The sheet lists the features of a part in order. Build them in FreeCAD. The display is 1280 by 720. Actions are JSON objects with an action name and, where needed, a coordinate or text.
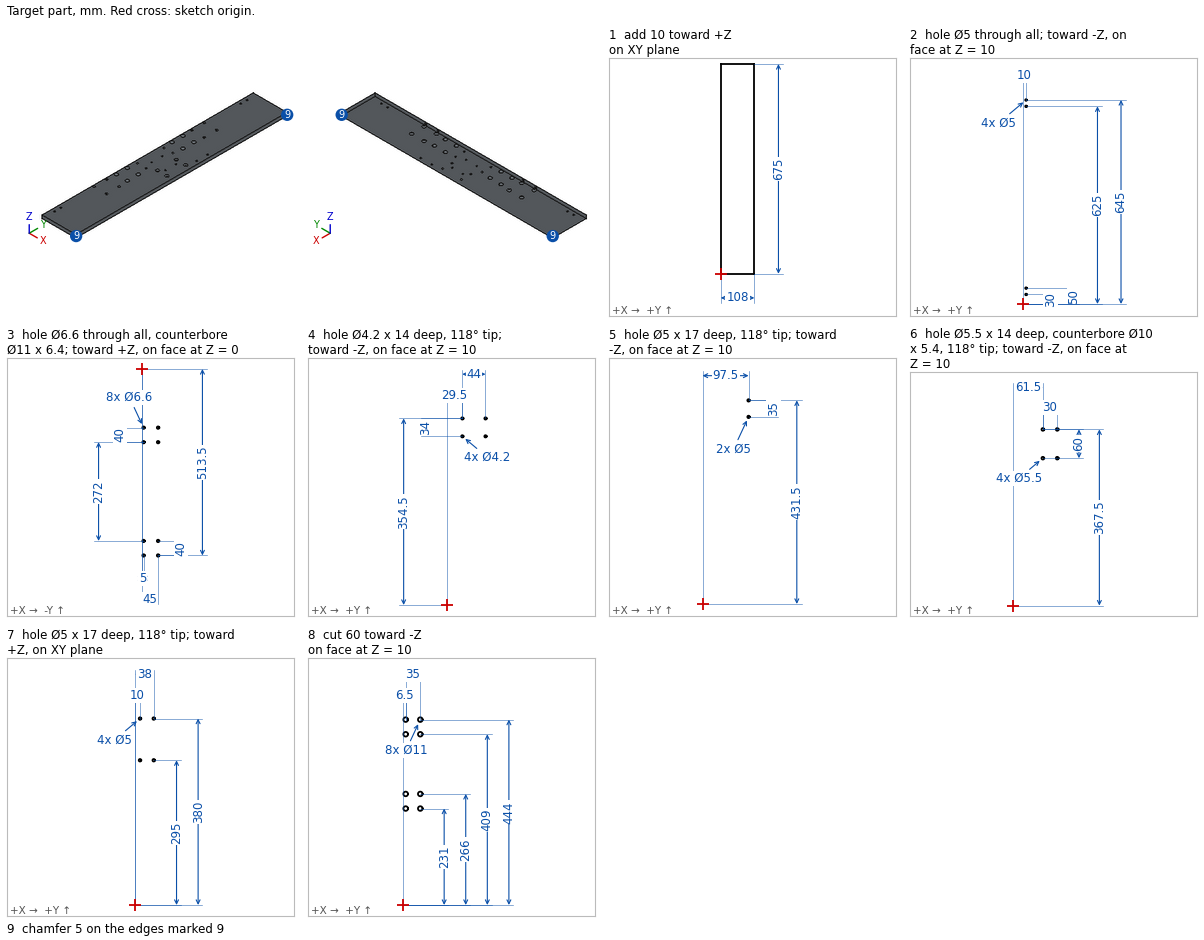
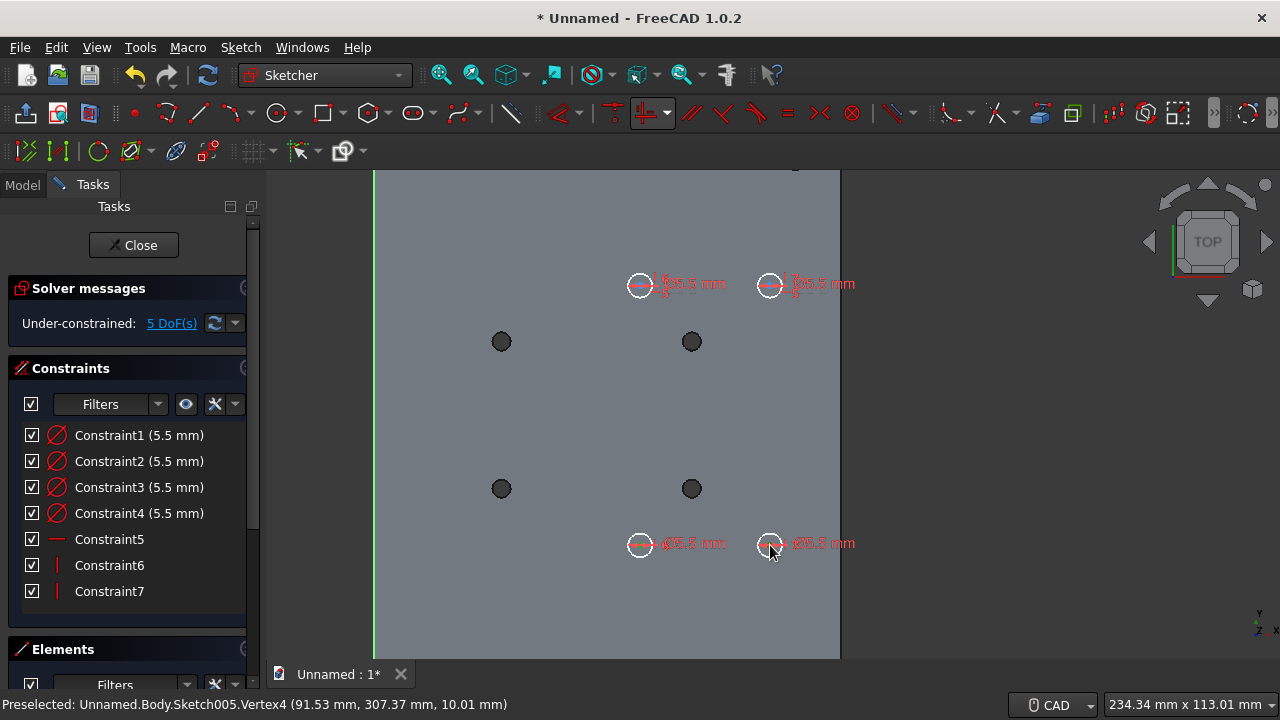
{"action": "key", "text": "h"}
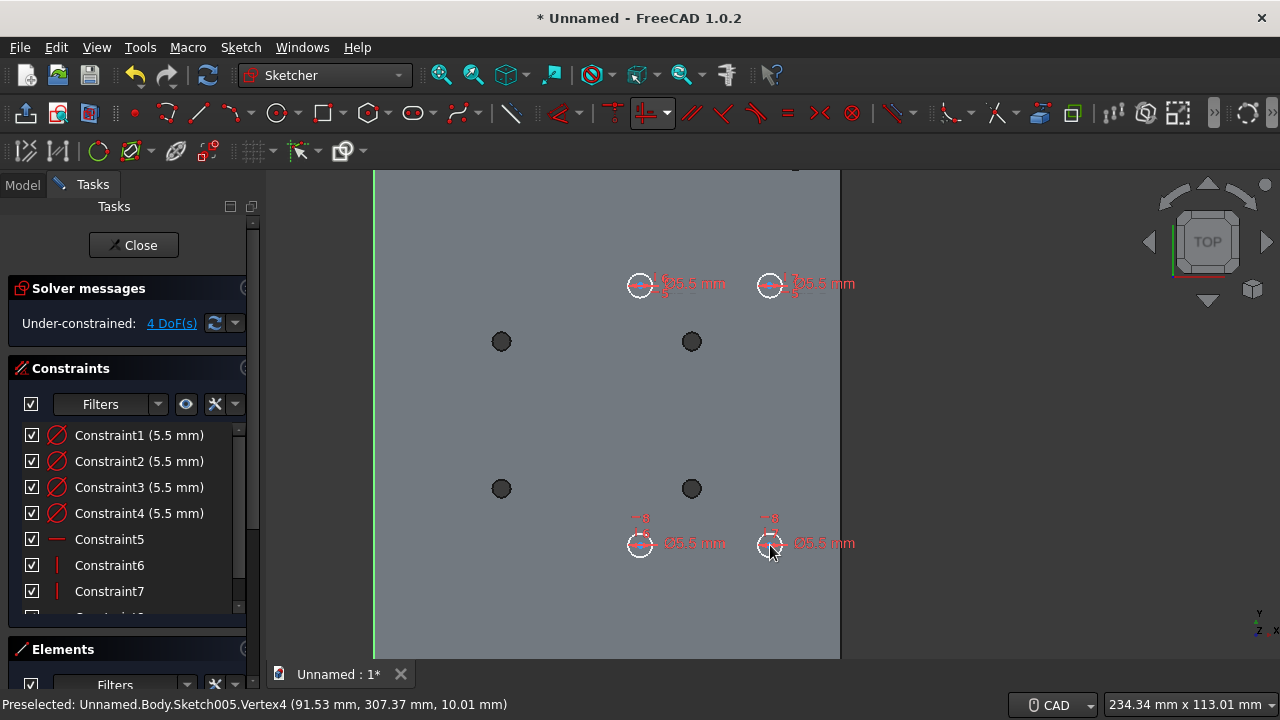
{"action": "left_click", "coordinate": [558, 114]}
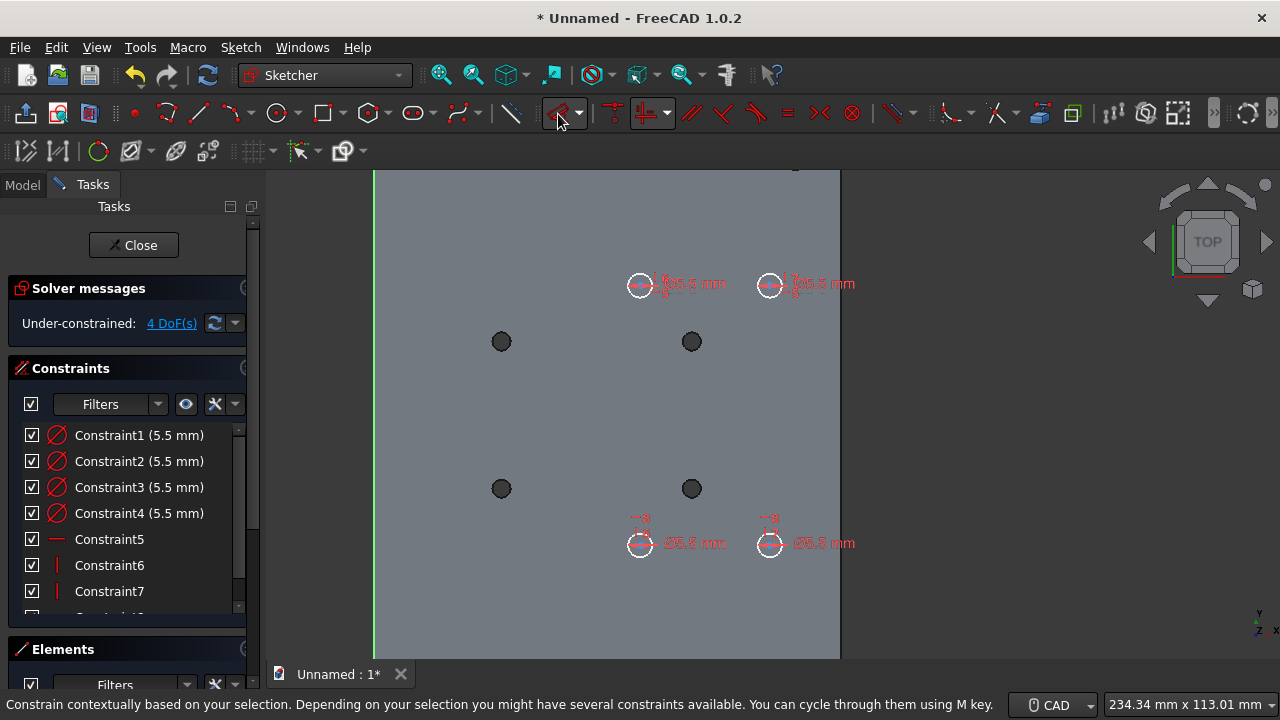
{"action": "left_click", "coordinate": [640, 286]}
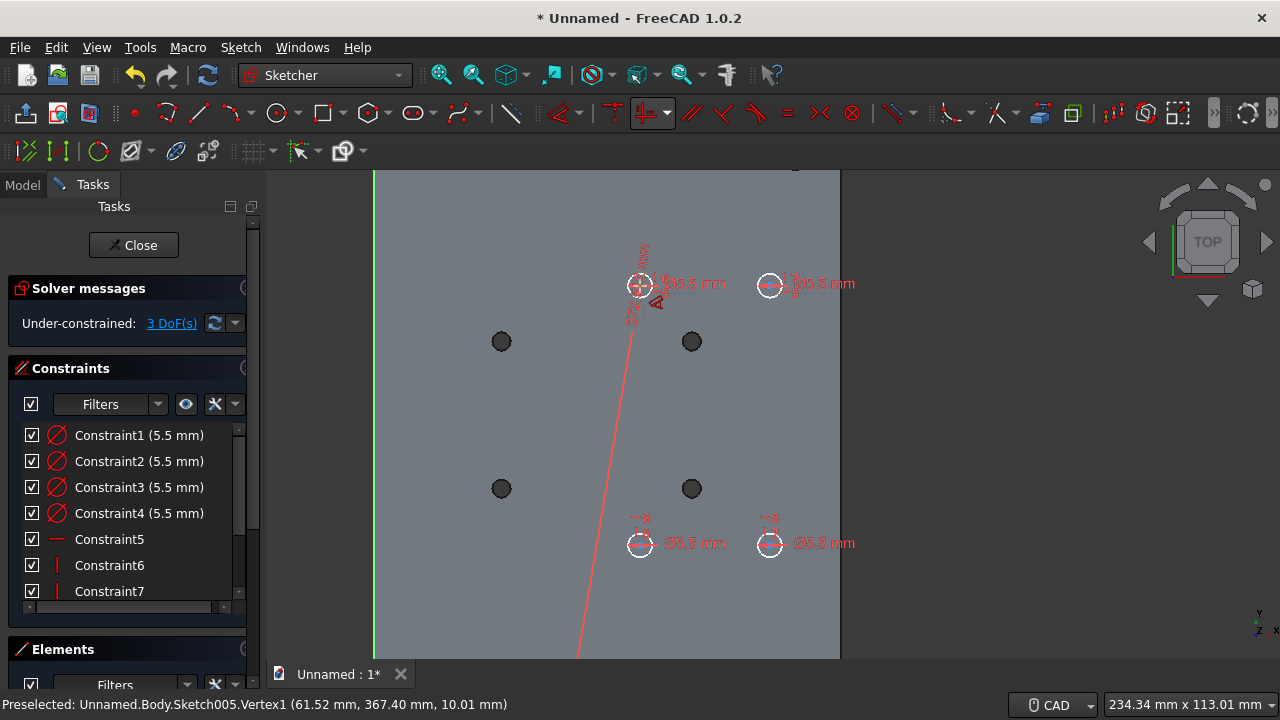
{"action": "left_click", "coordinate": [770, 286]}
{"action": "left_click", "coordinate": [705, 252]}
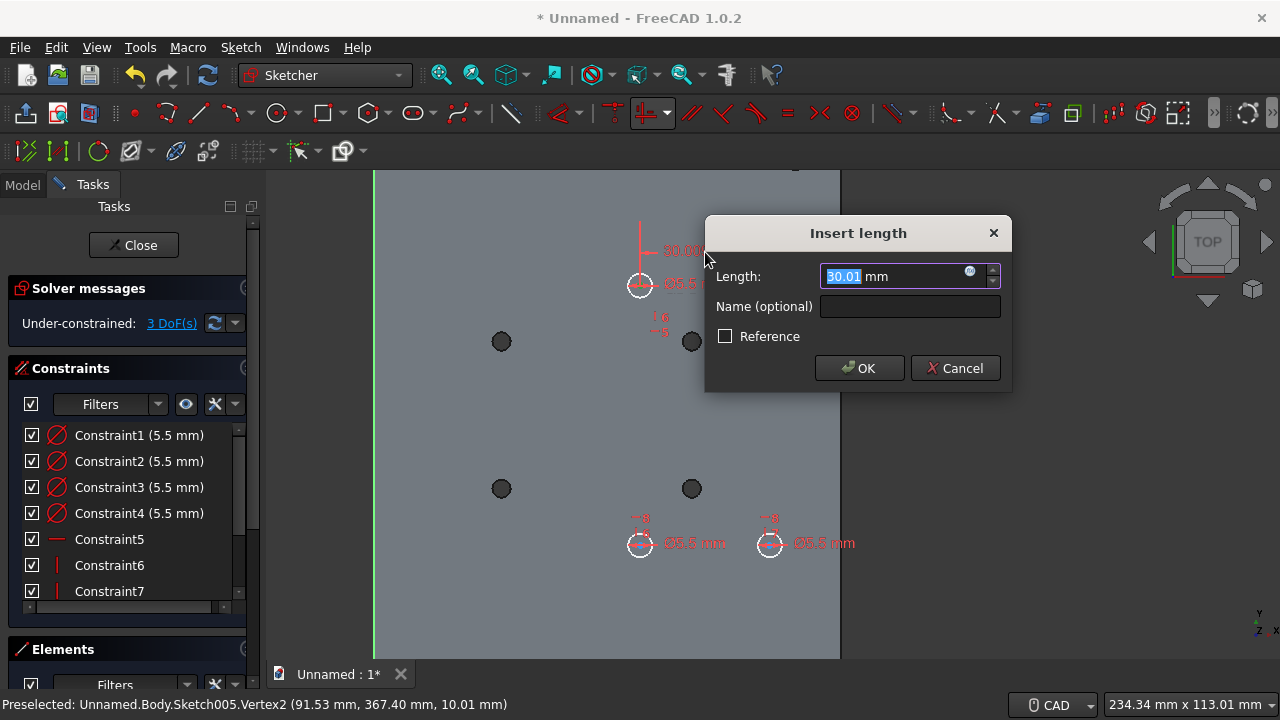
{"action": "type", "text": "30"}
{"action": "key", "text": "Return"}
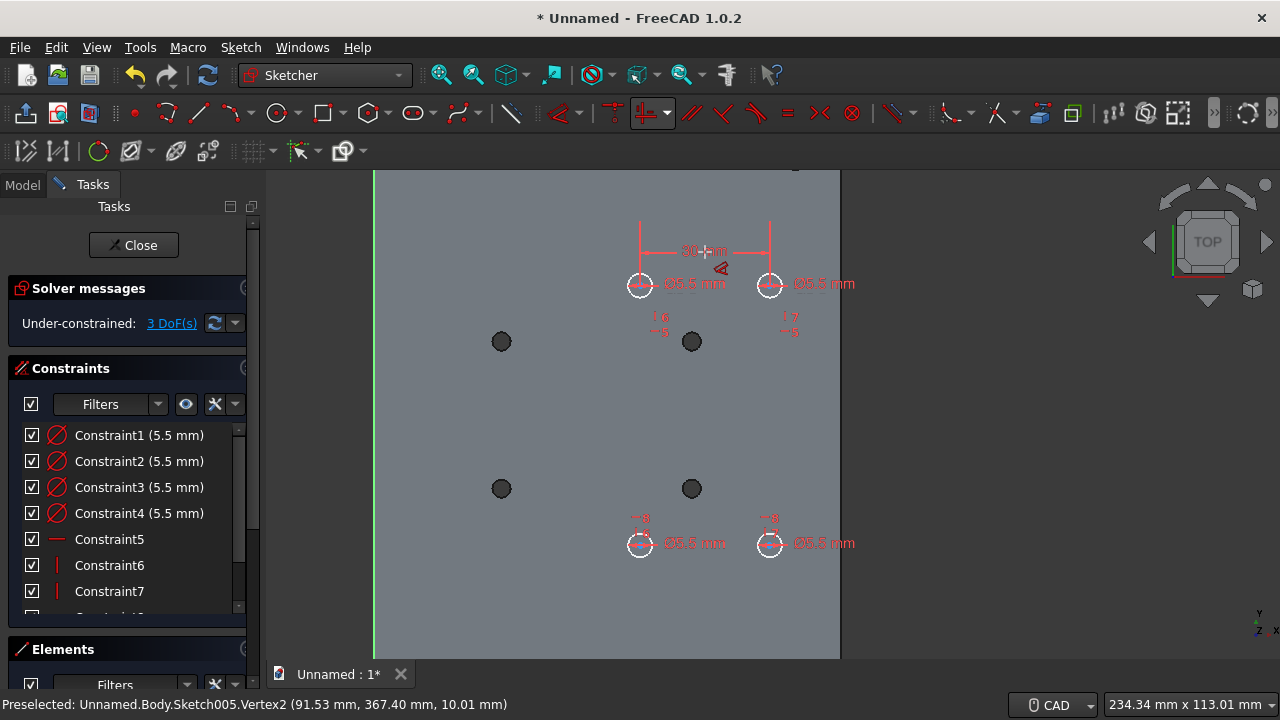
{"action": "left_click", "coordinate": [640, 286]}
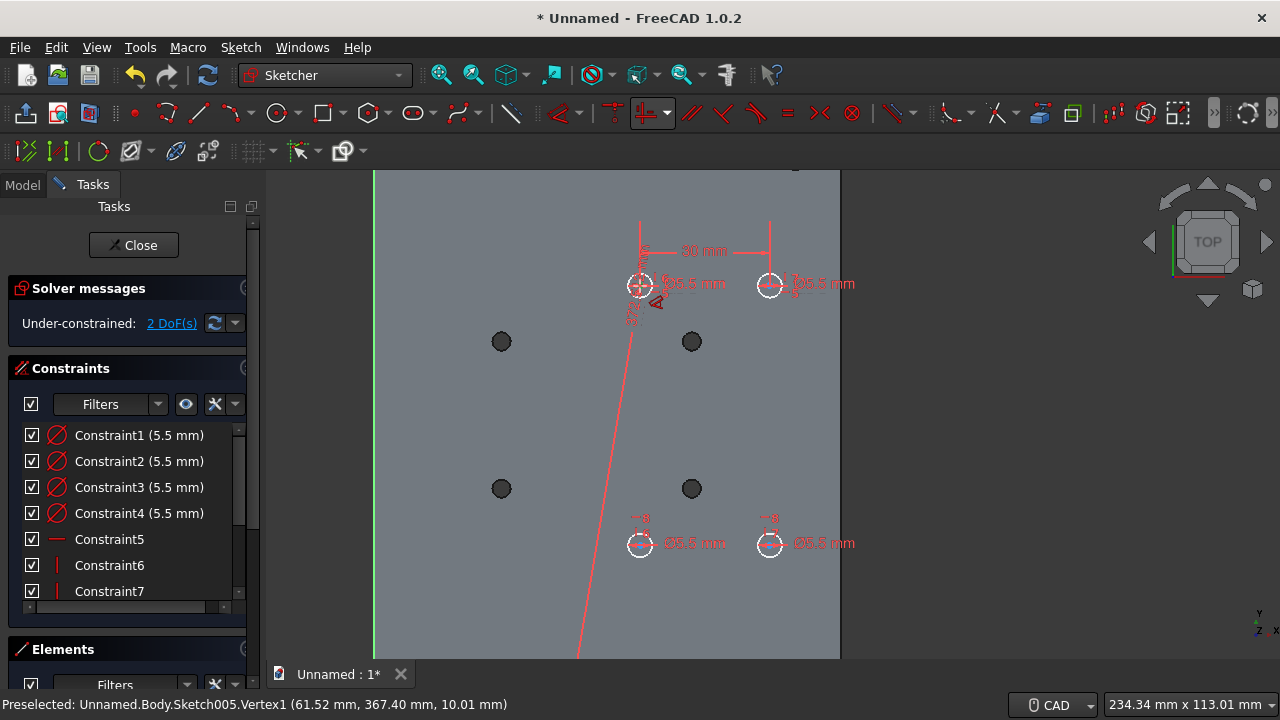
{"action": "left_click", "coordinate": [640, 545]}
{"action": "left_click", "coordinate": [606, 416]}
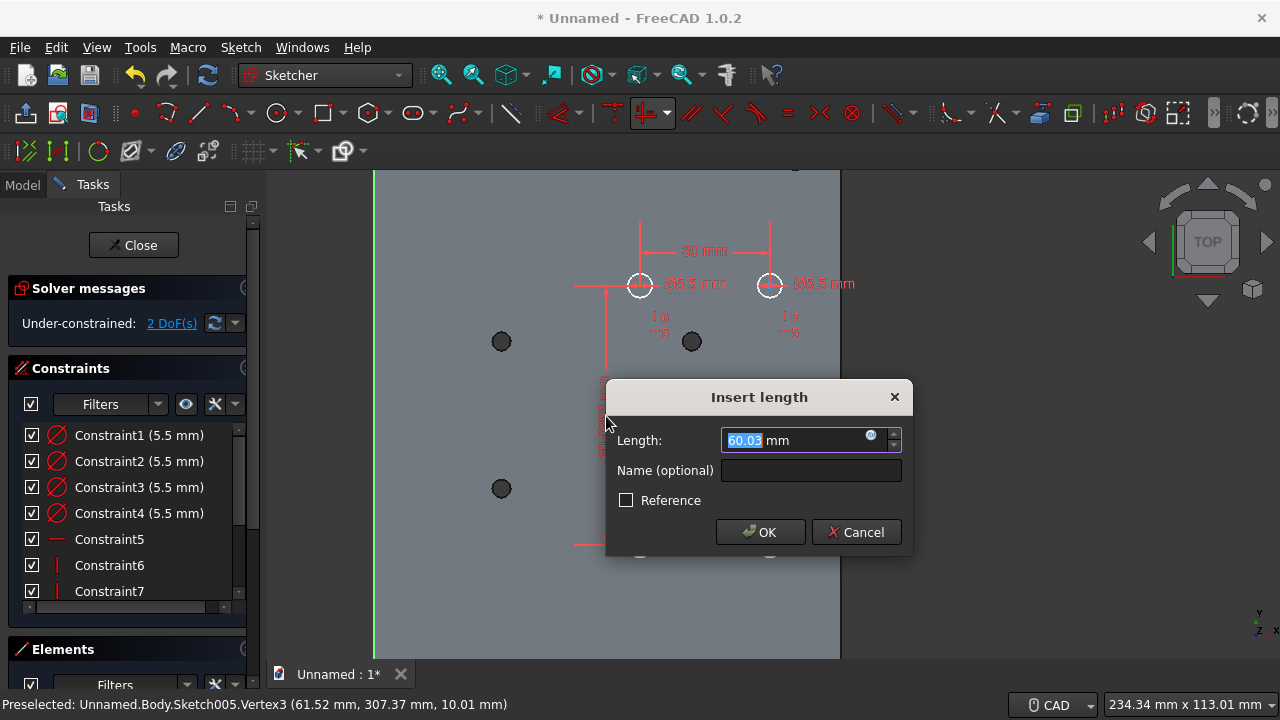
{"action": "type", "text": "60"}
{"action": "key", "text": "Return"}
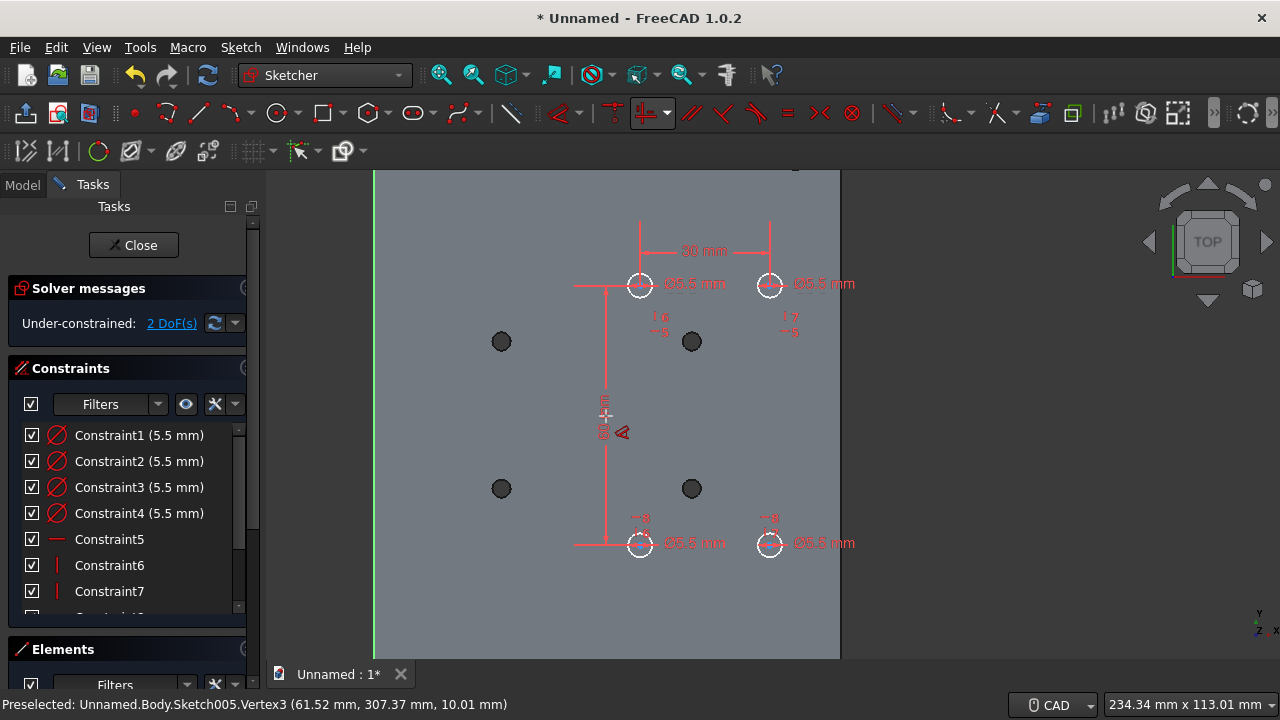
{"action": "left_click", "coordinate": [640, 286]}
{"action": "left_click", "coordinate": [507, 252]}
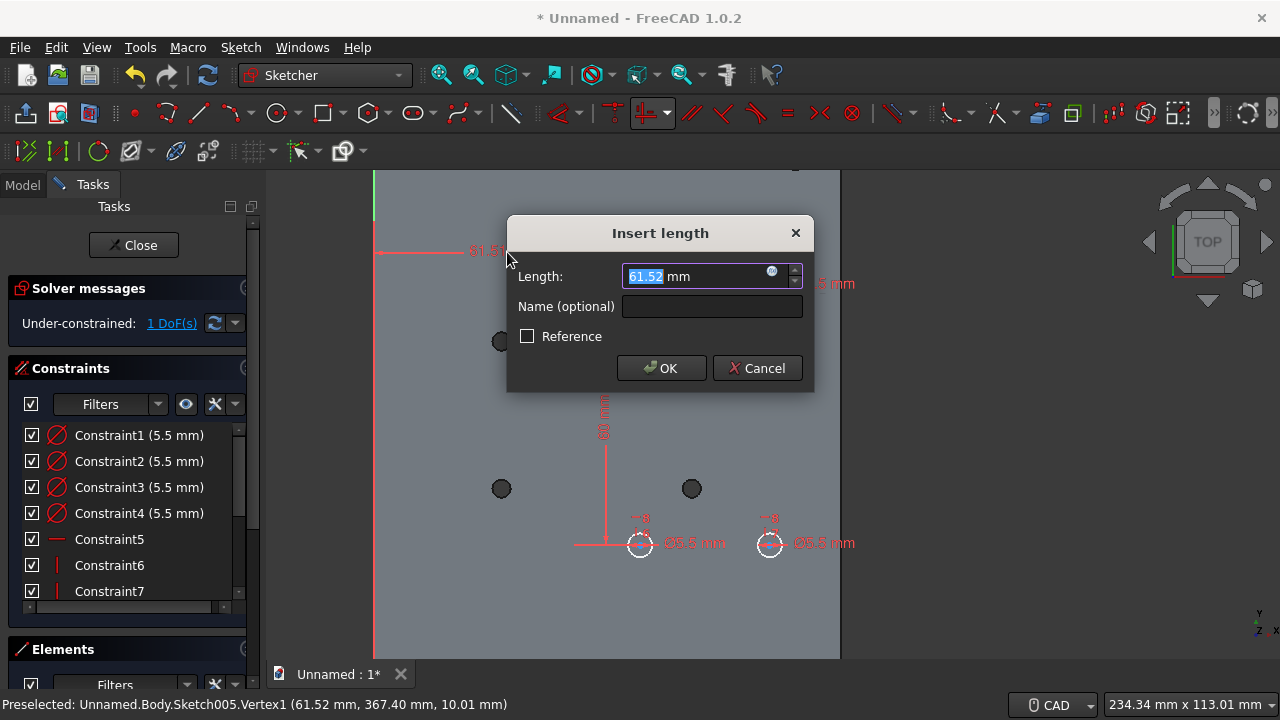
{"action": "type", "text": "61.5"}
{"action": "key", "text": "Return"}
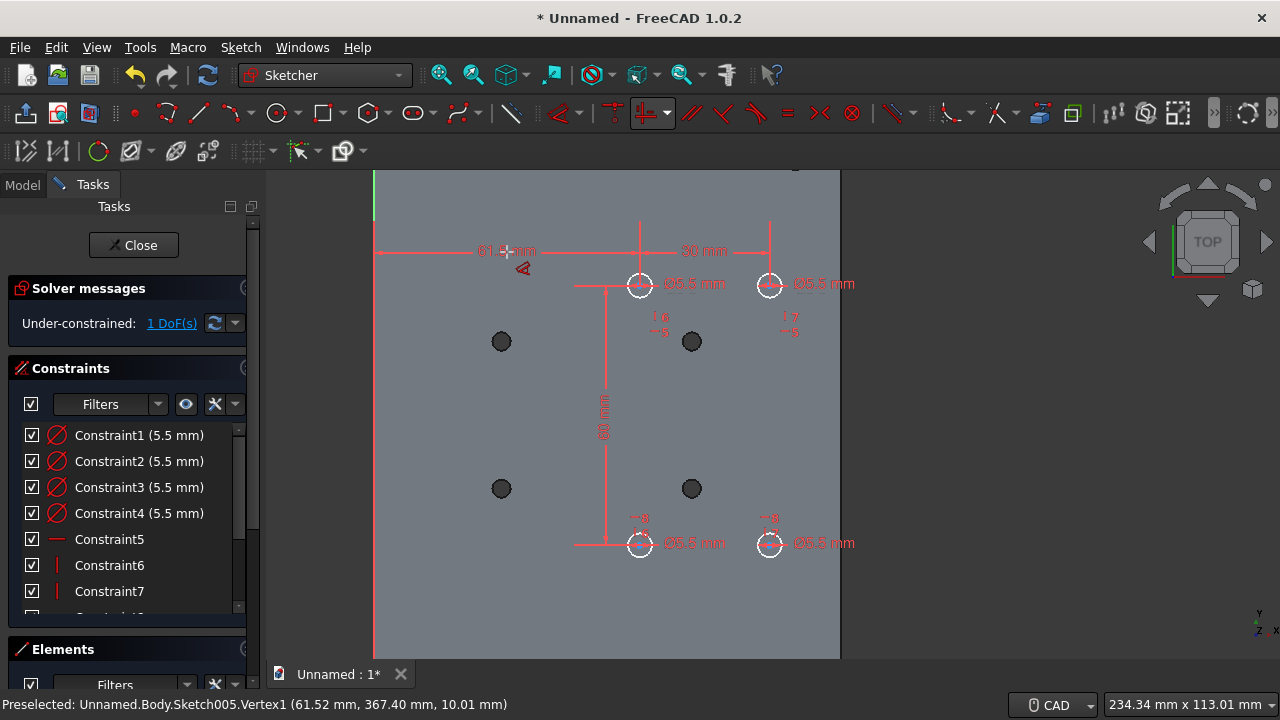
{"action": "left_click", "coordinate": [640, 286]}
{"action": "left_click", "coordinate": [340, 458]}